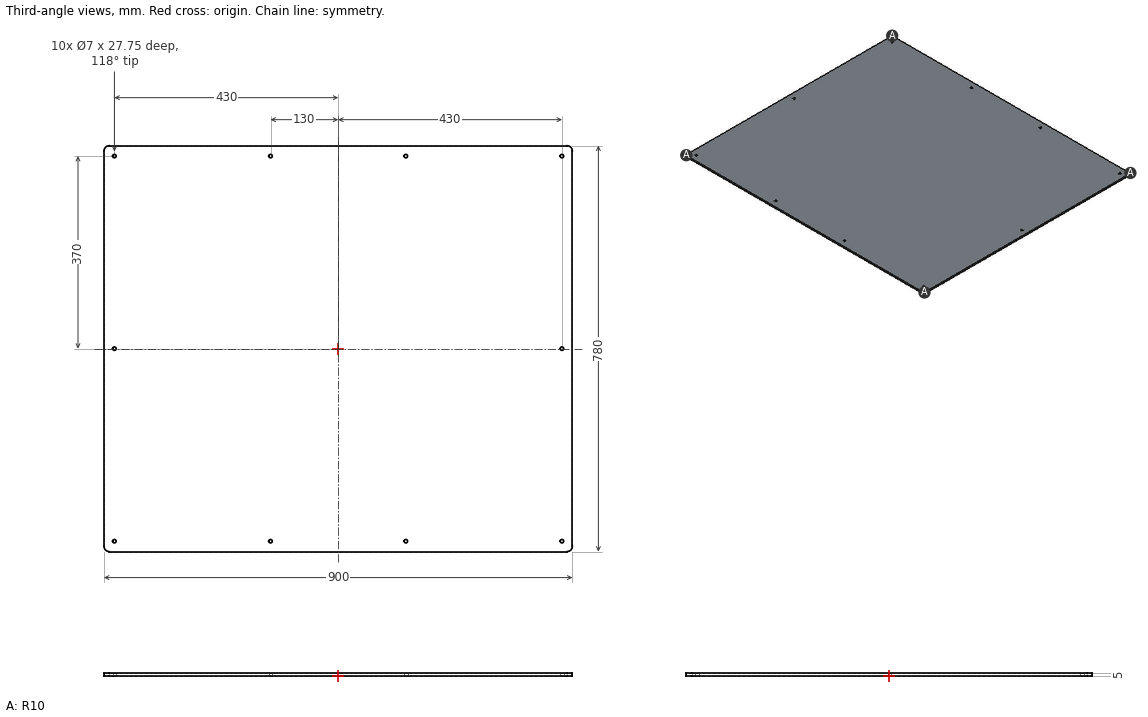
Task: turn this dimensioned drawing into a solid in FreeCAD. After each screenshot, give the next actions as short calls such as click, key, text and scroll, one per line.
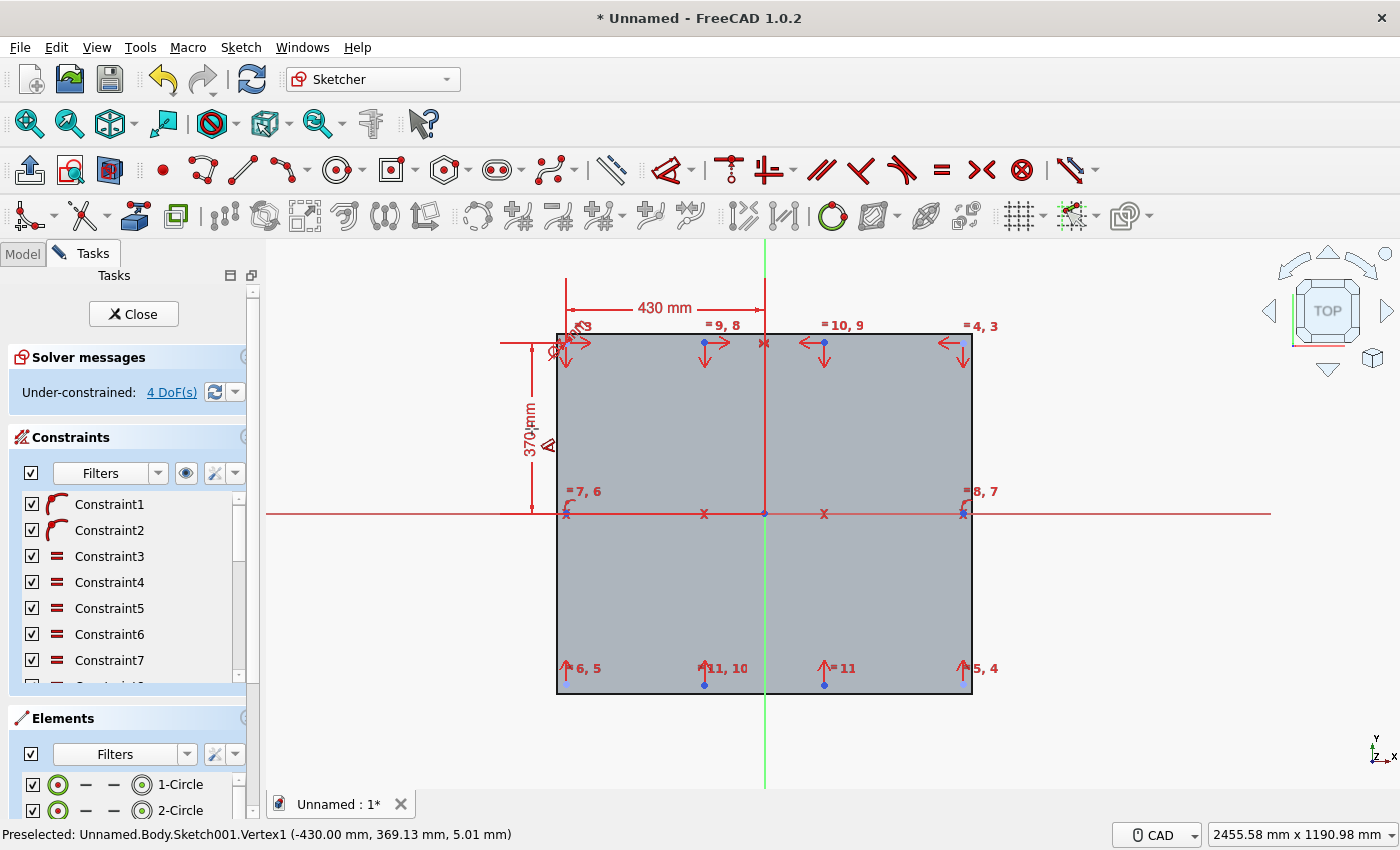
click(566, 514)
click(665, 548)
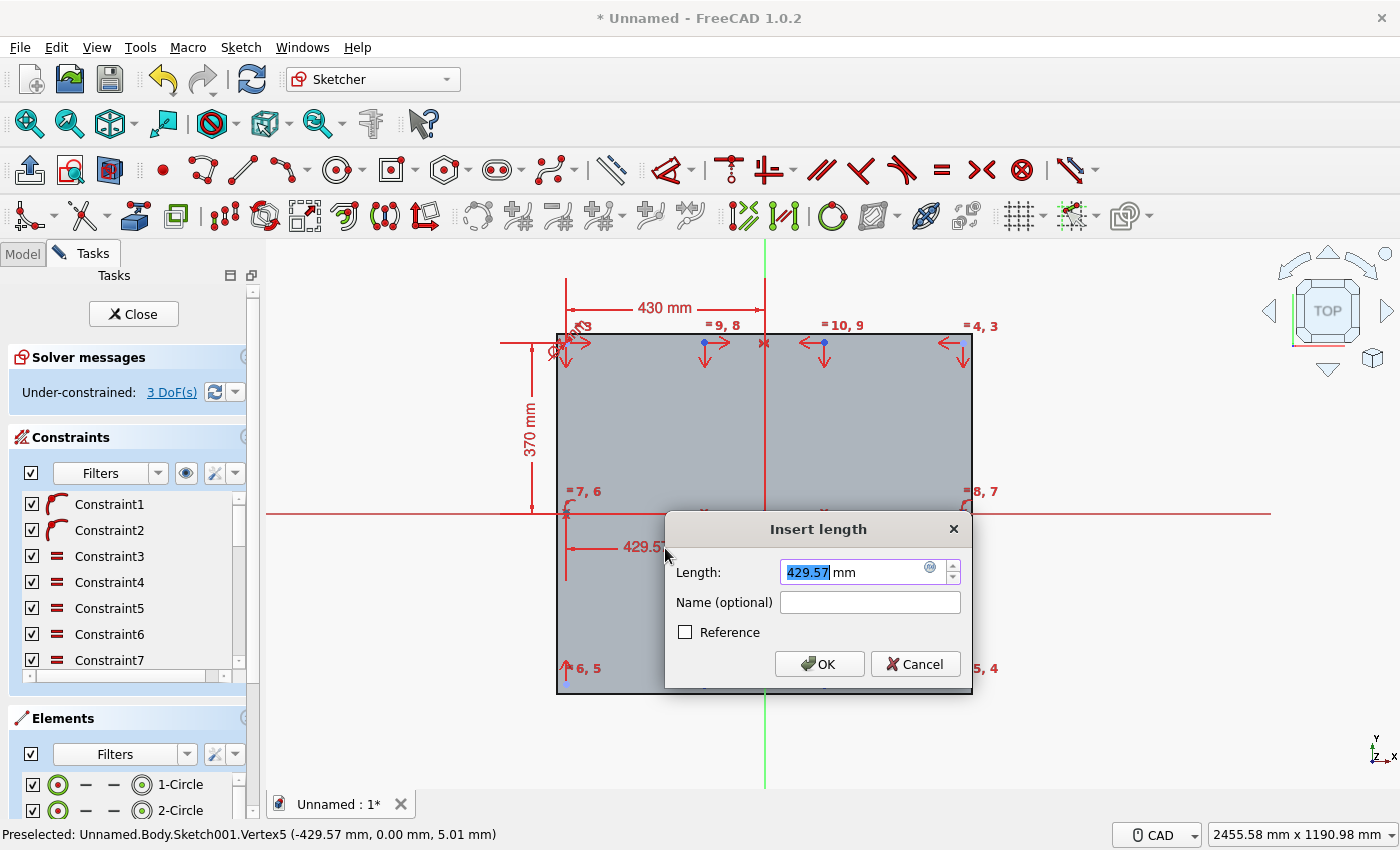
text(430)
key(Return)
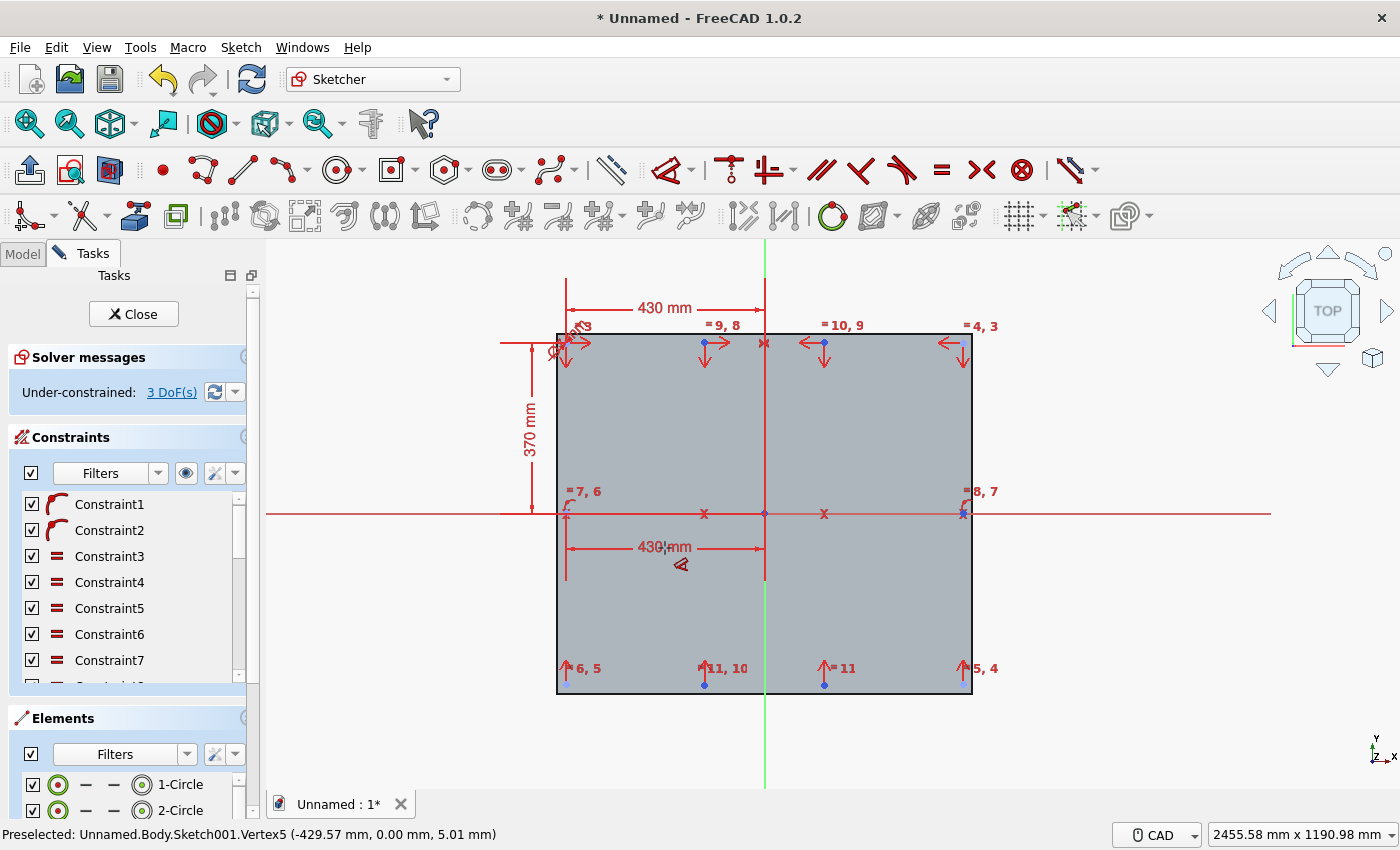
click(963, 514)
click(864, 548)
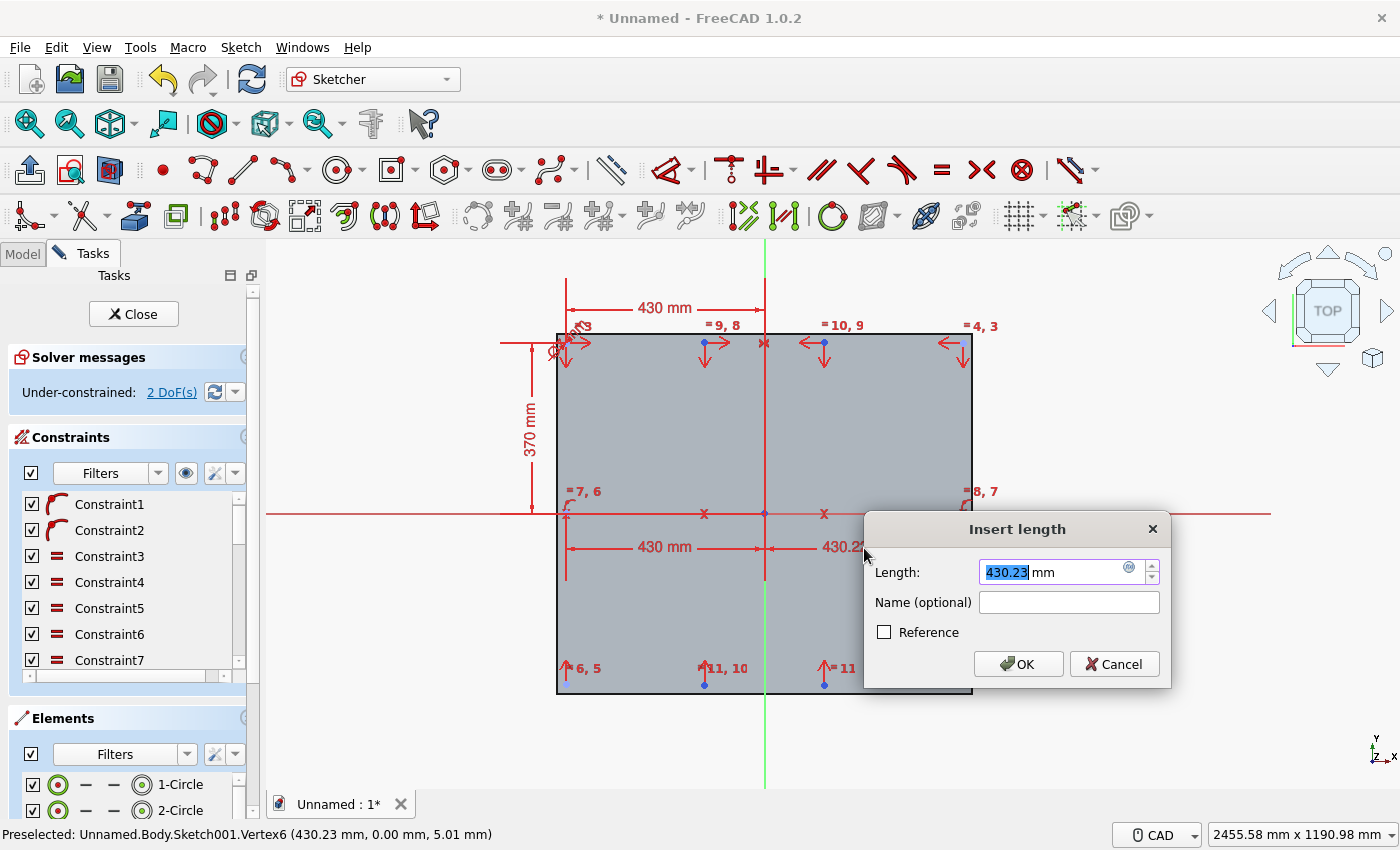
text(430)
key(Return)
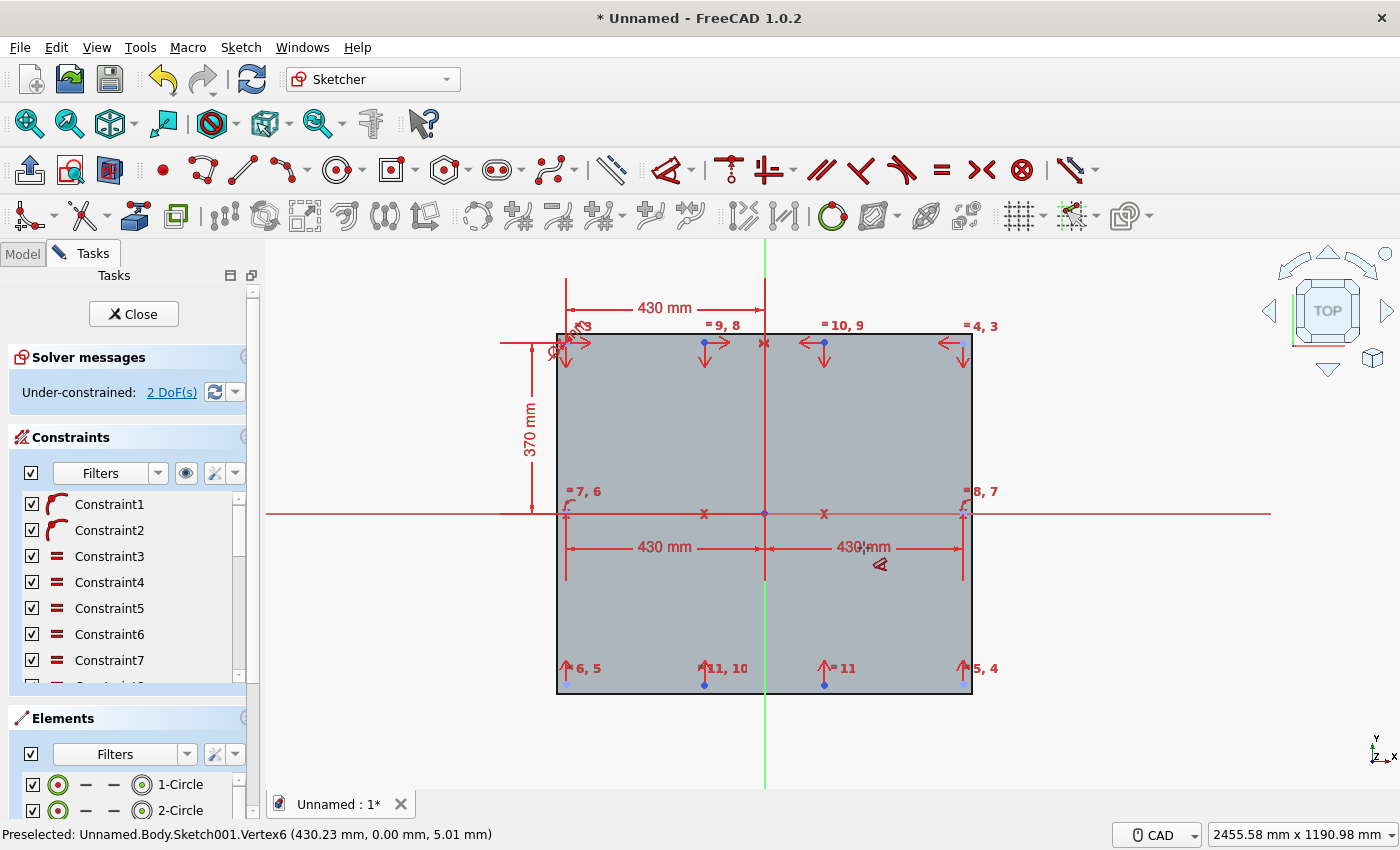
click(705, 343)
click(748, 309)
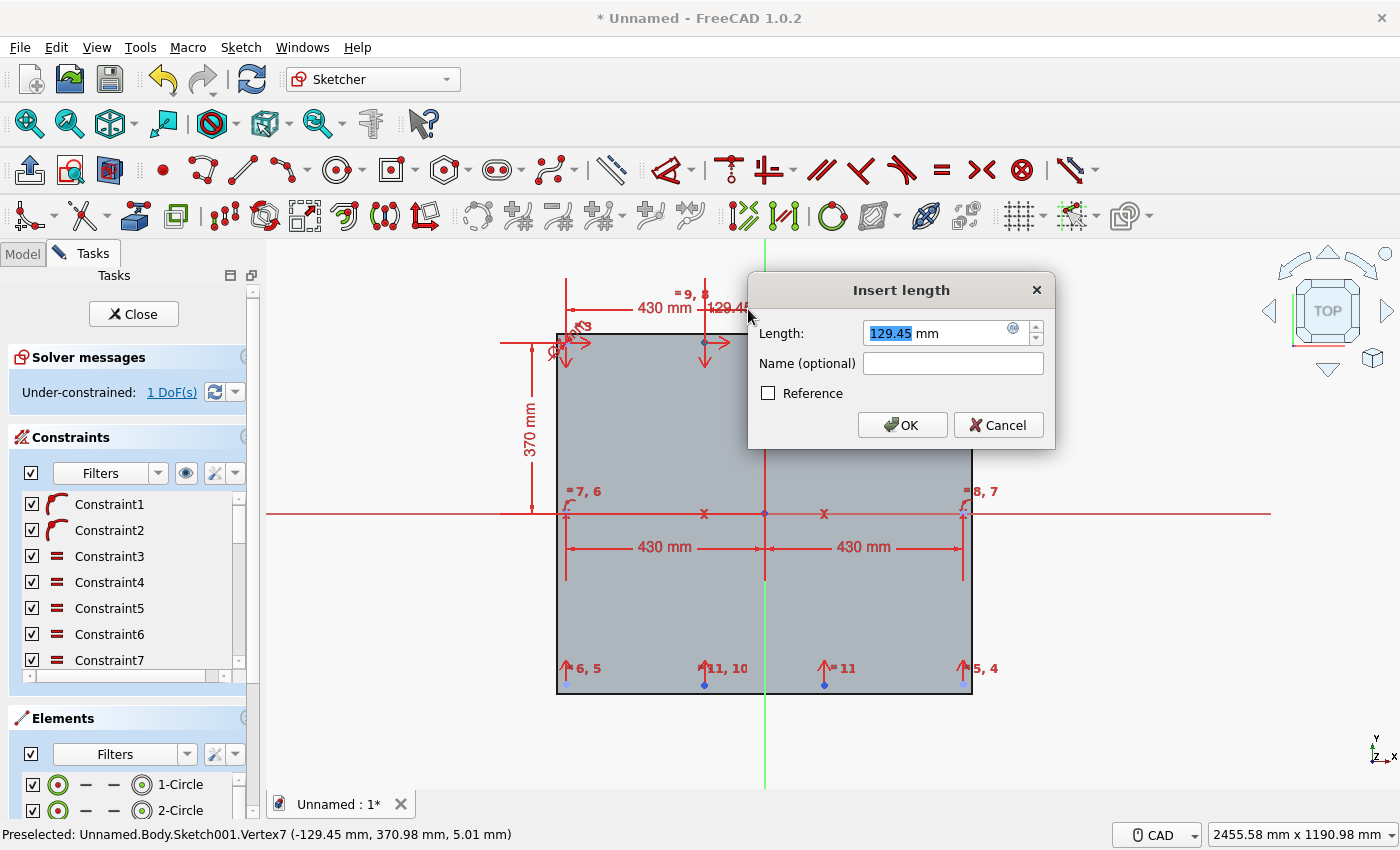
text(130)
key(Return)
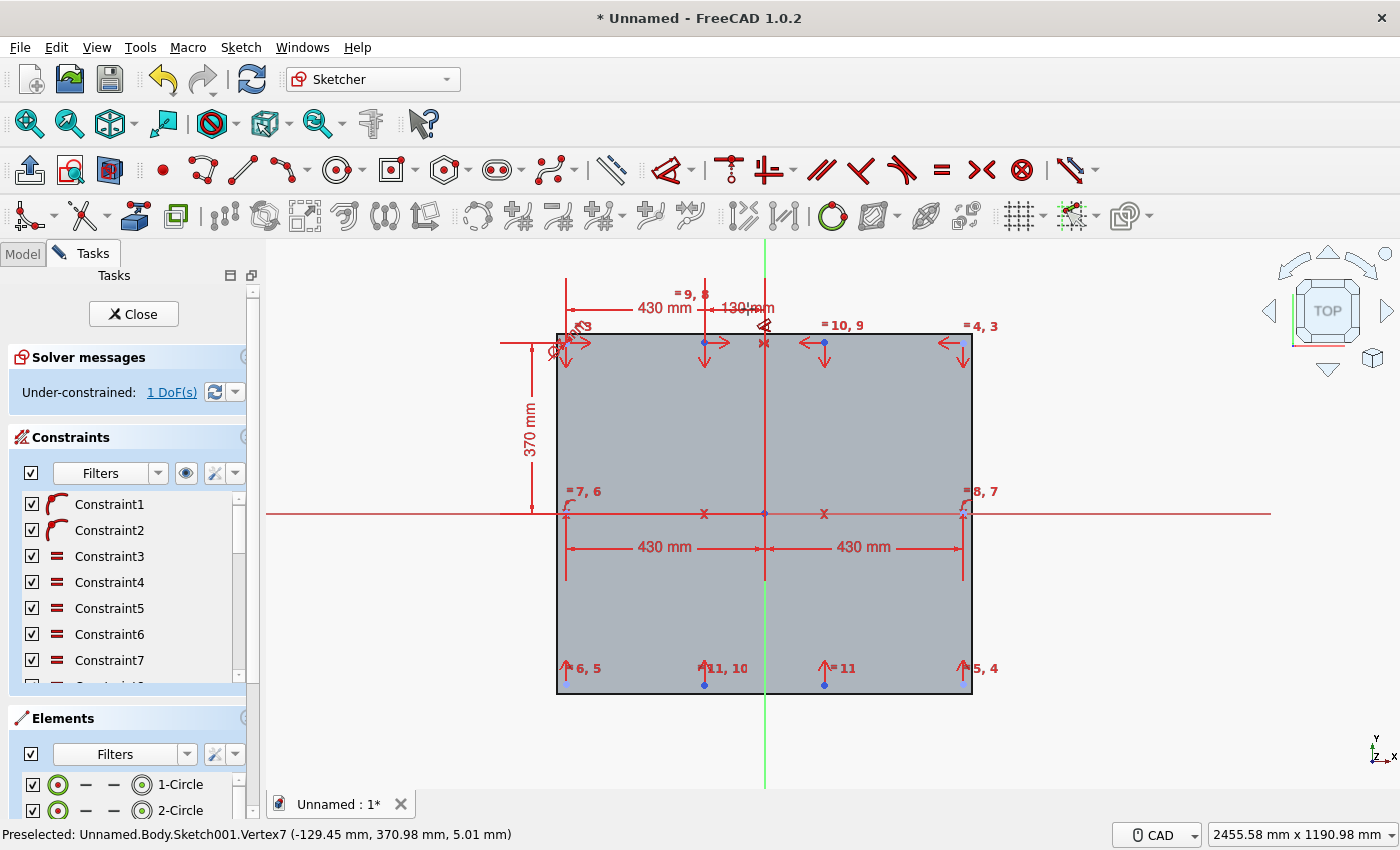
click(705, 343)
click(671, 428)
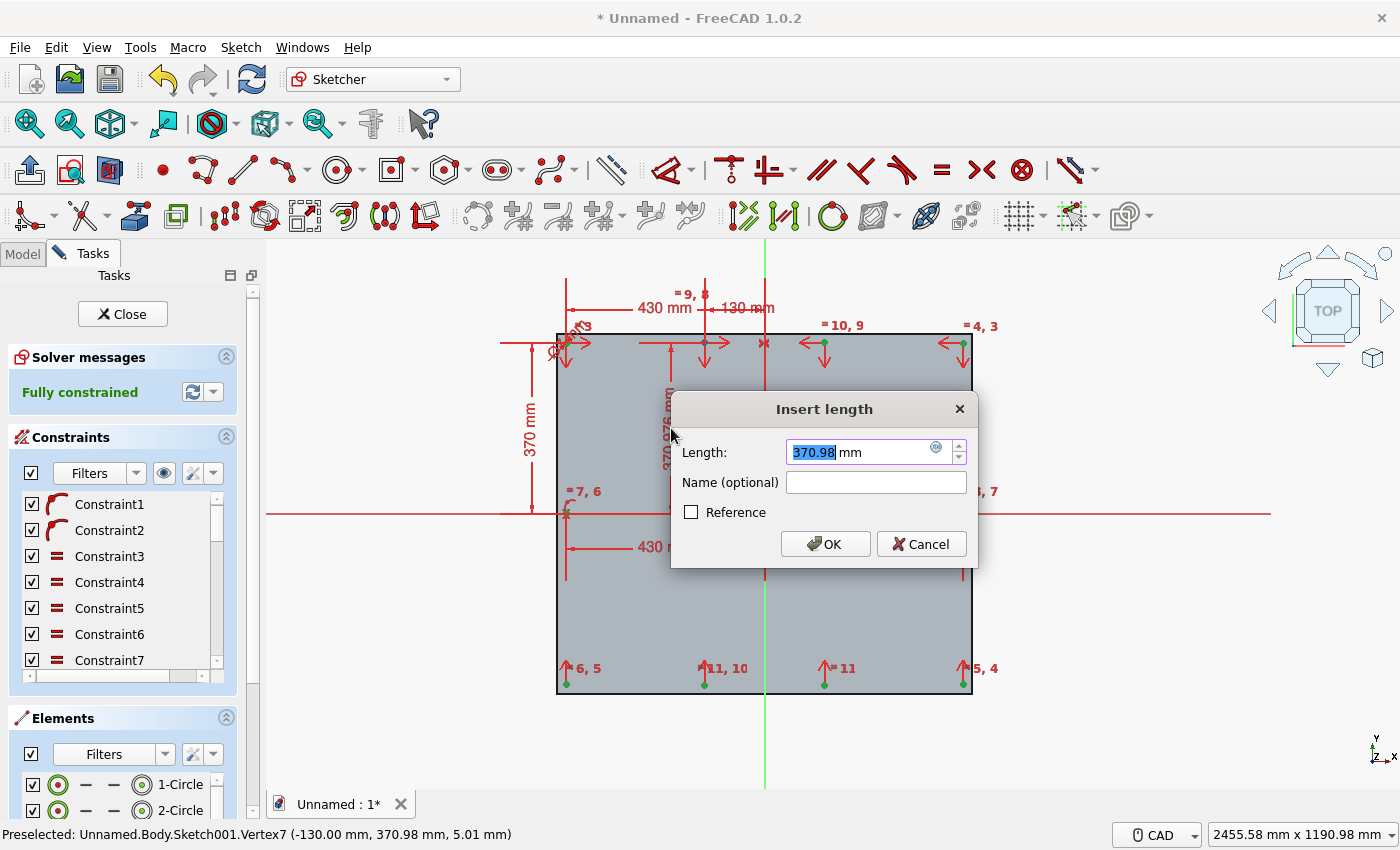
text(370)
key(Return)
key(Escape)